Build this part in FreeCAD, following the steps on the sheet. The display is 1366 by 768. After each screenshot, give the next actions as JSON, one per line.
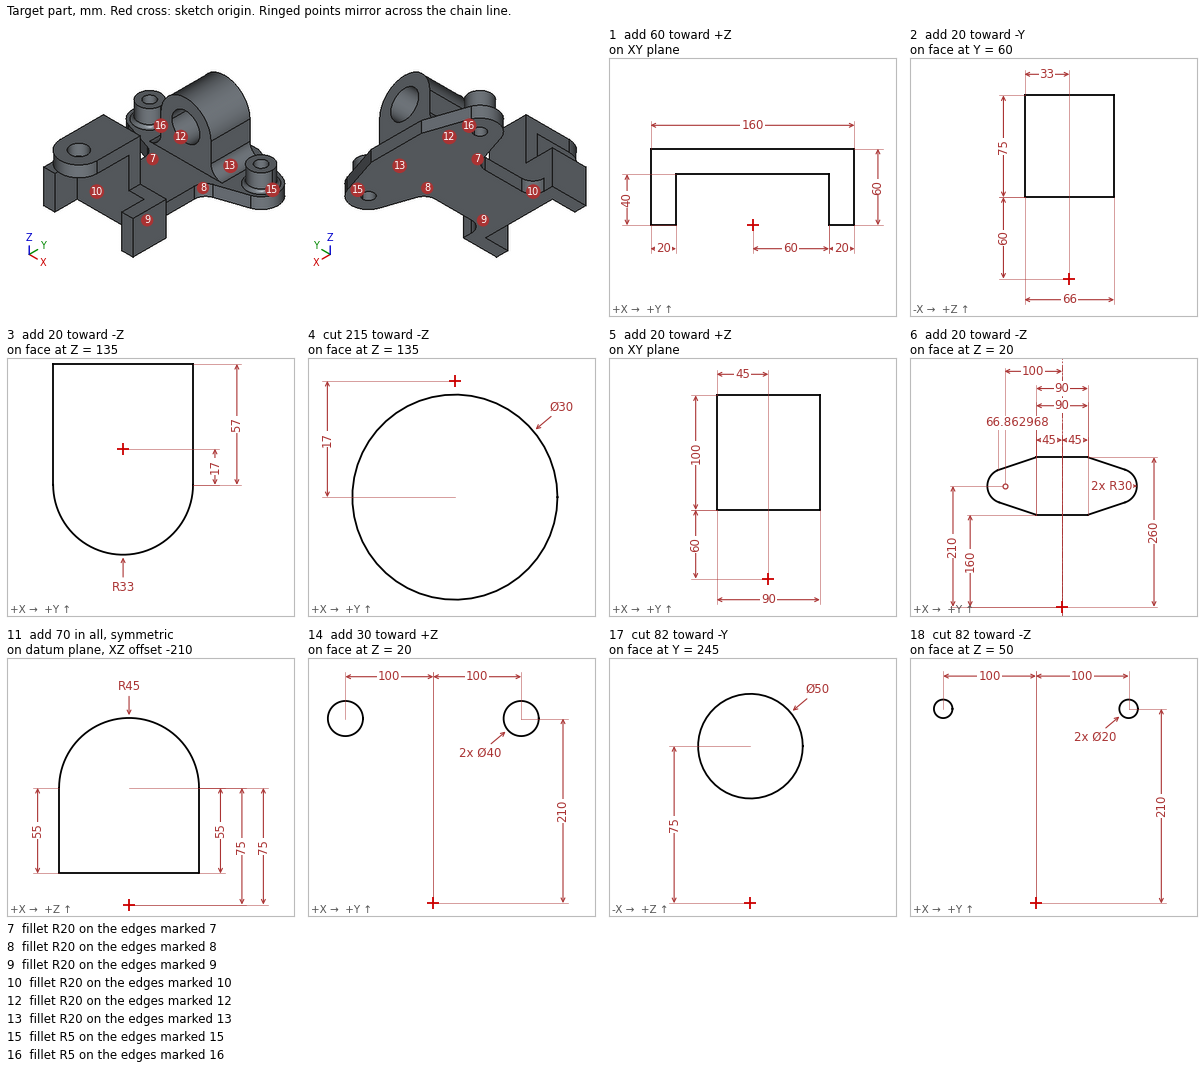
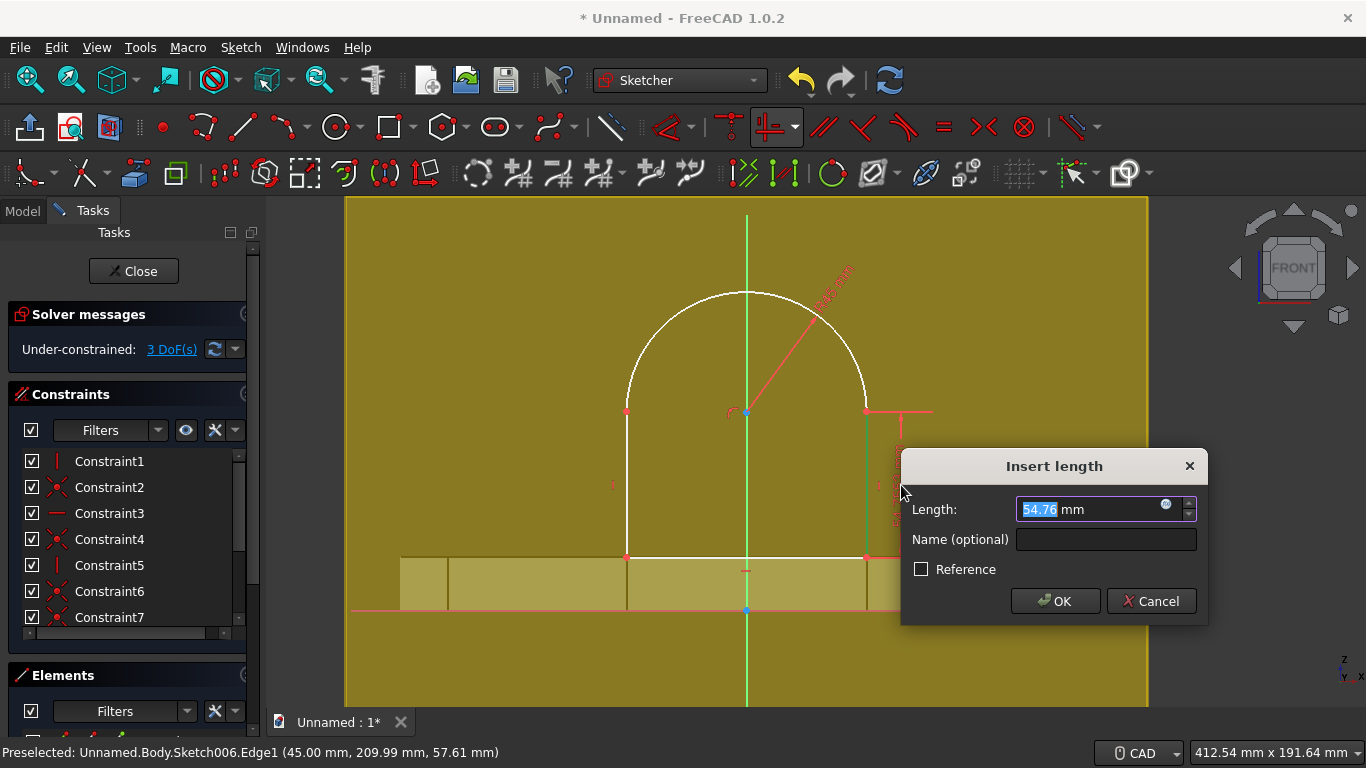
{"action": "type", "text": "55"}
{"action": "key", "text": "Return"}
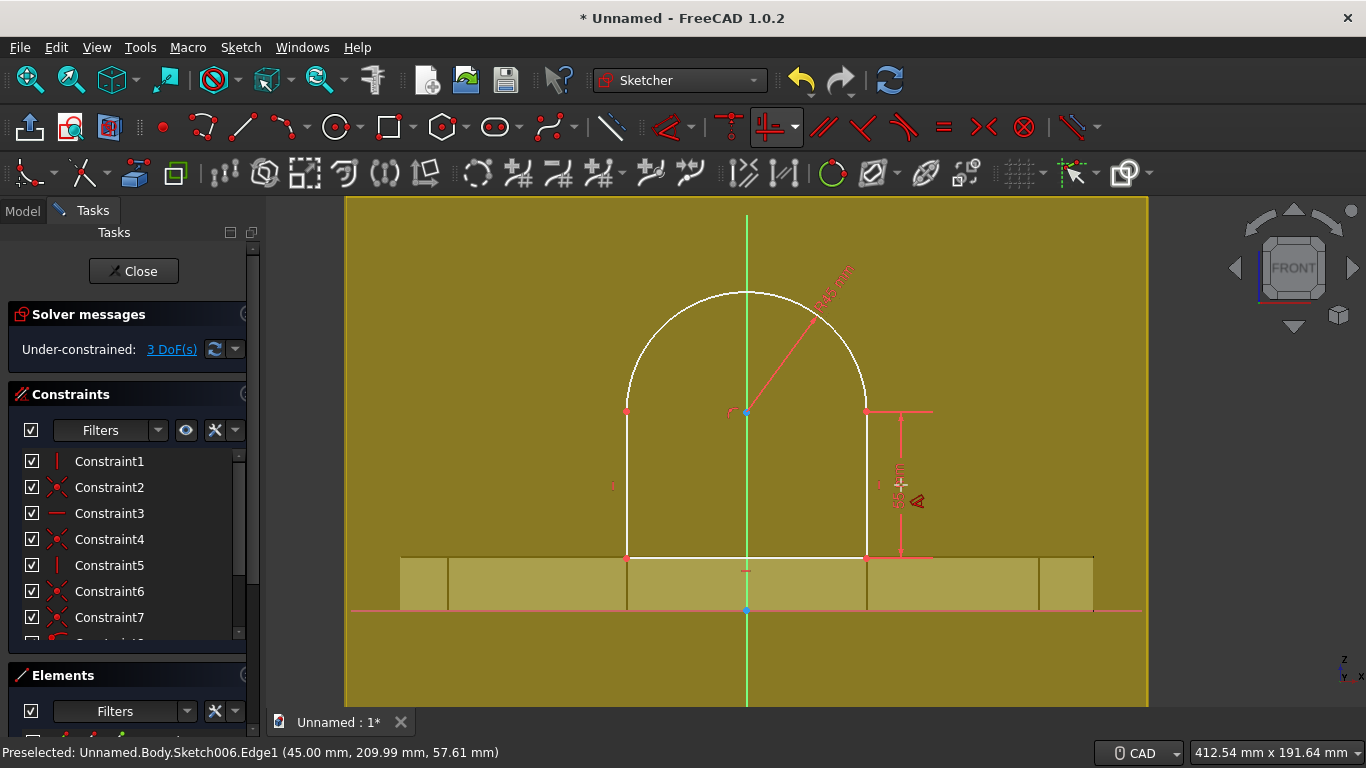
{"action": "left_click", "coordinate": [627, 514]}
{"action": "left_click", "coordinate": [593, 485]}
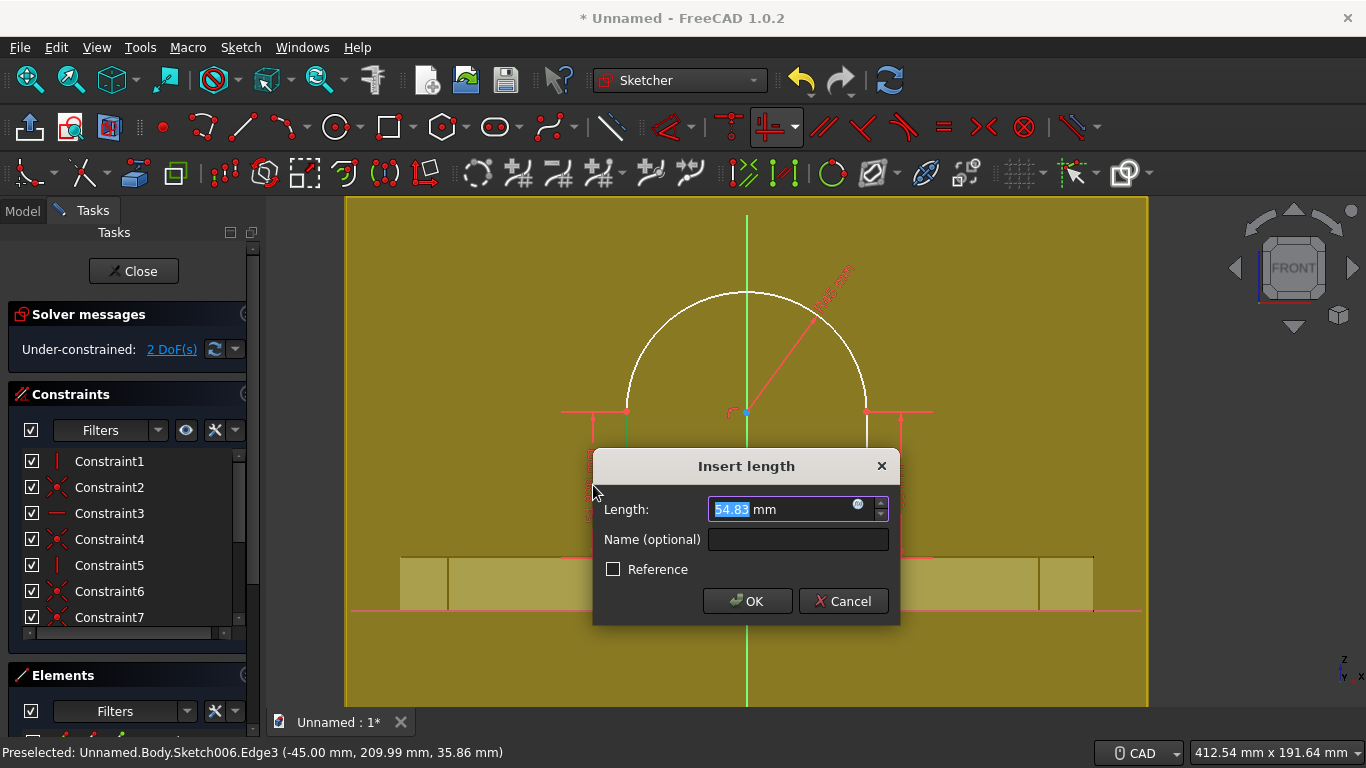
{"action": "type", "text": "55"}
{"action": "key", "text": "Return"}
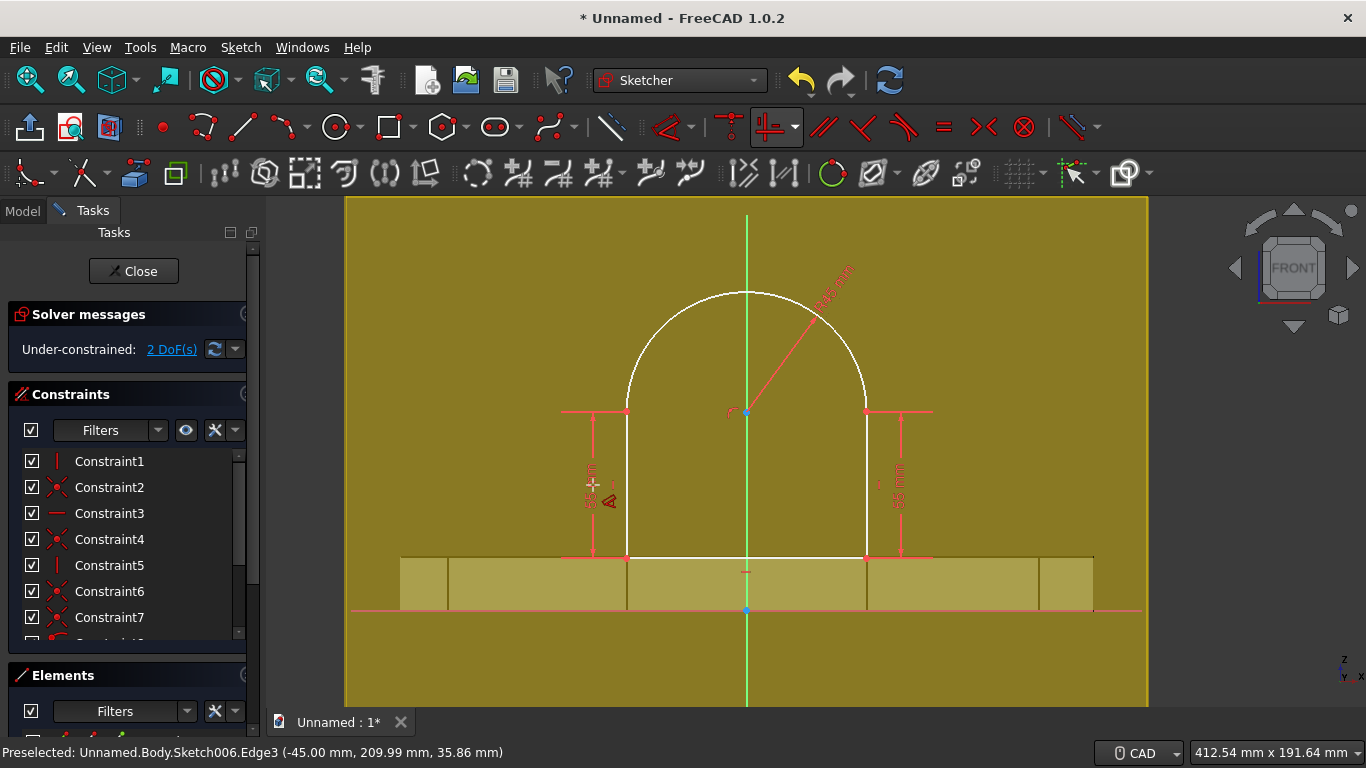
{"action": "left_click", "coordinate": [867, 412]}
{"action": "left_click", "coordinate": [901, 511]}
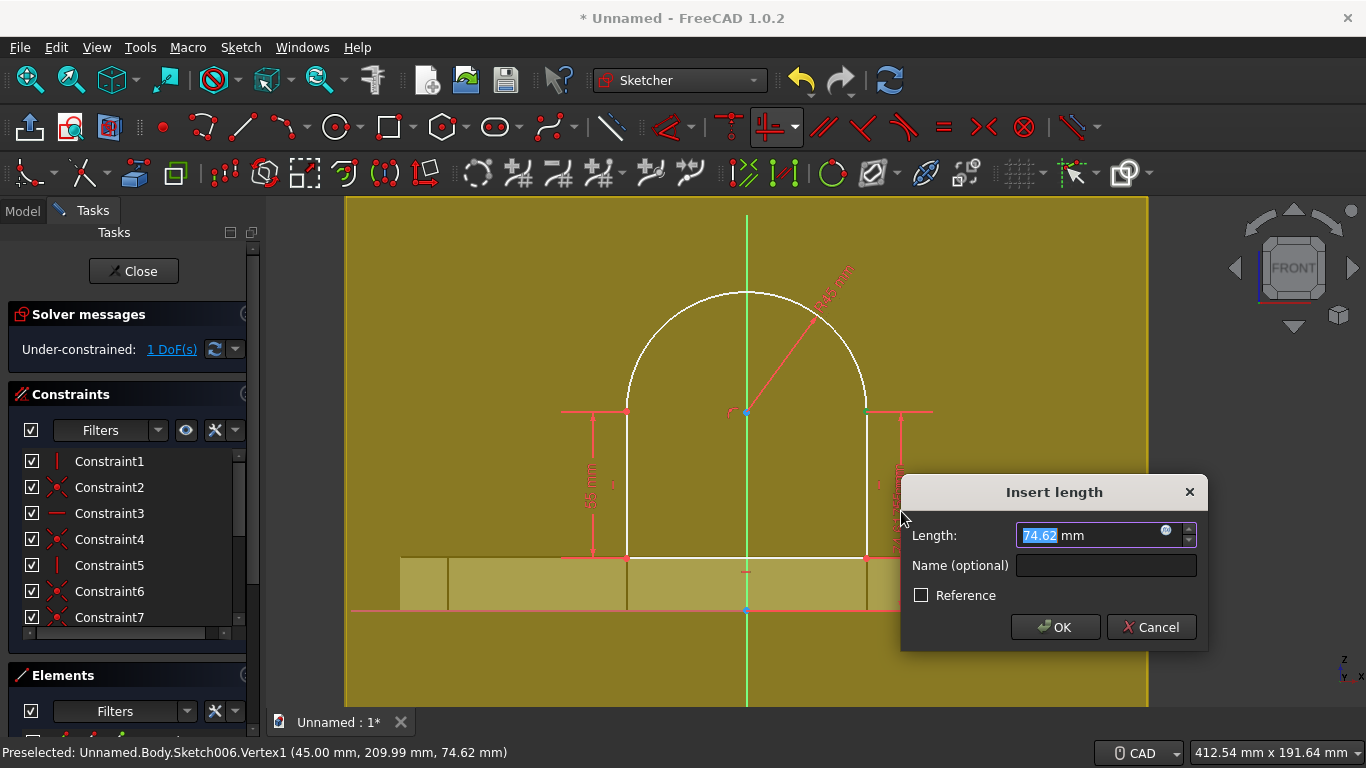
{"action": "type", "text": "75"}
{"action": "key", "text": "Return"}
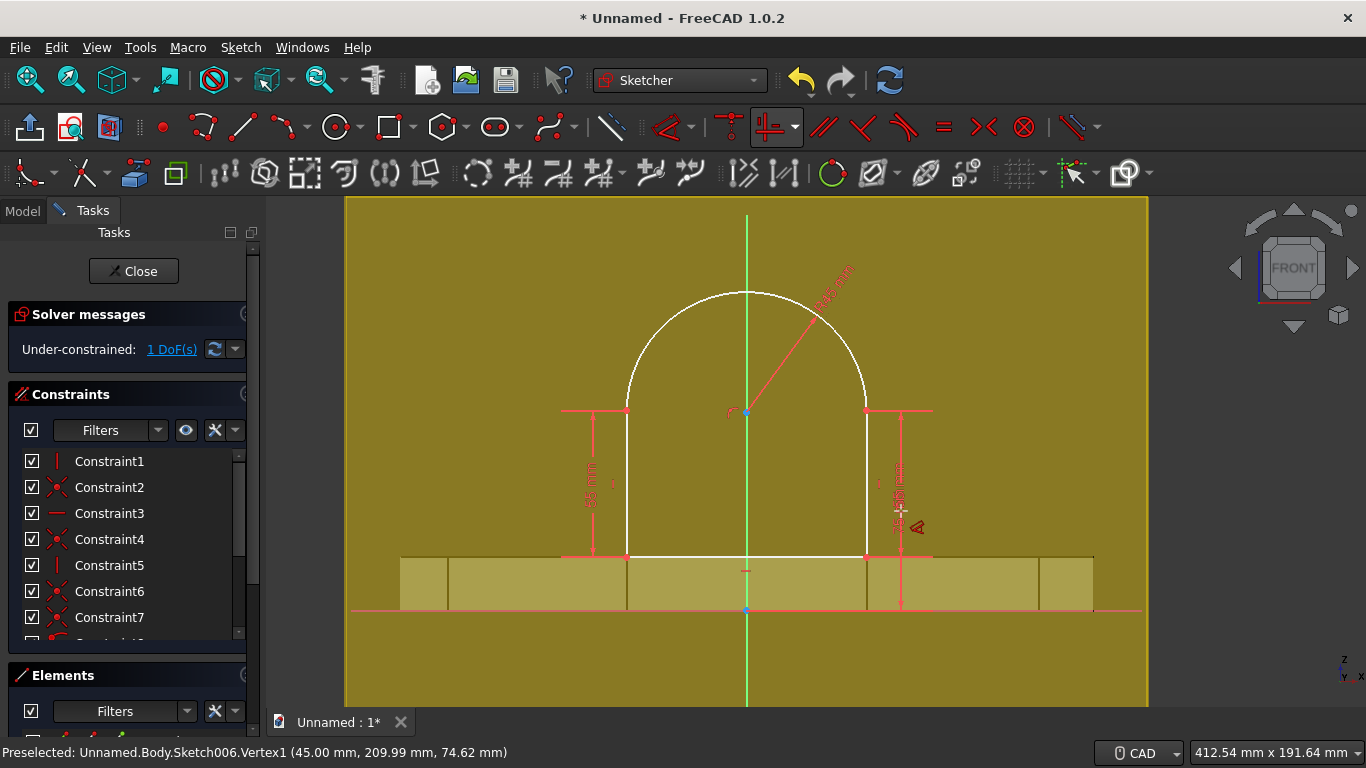
{"action": "left_click", "coordinate": [747, 412]}
{"action": "left_click", "coordinate": [781, 511]}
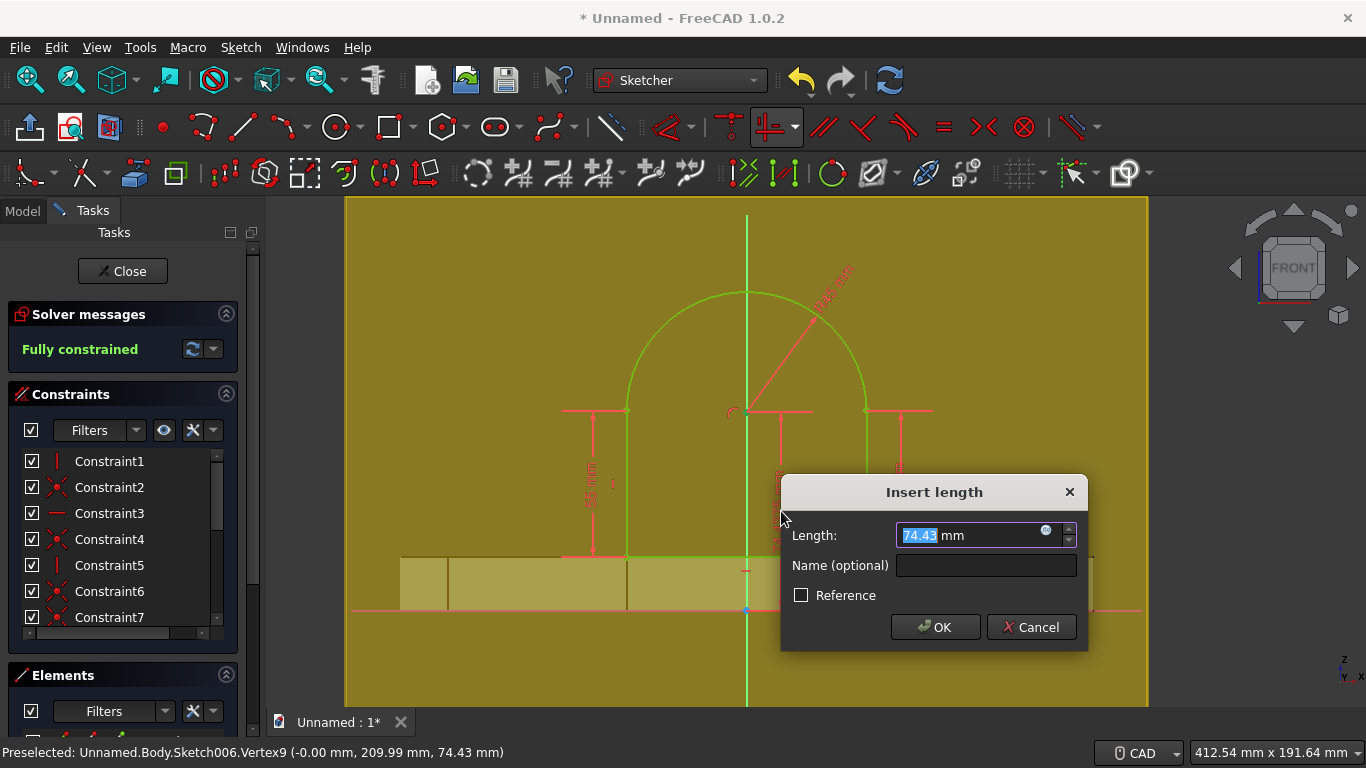
{"action": "type", "text": "75"}
{"action": "key", "text": "Return"}
{"action": "key", "text": "Escape"}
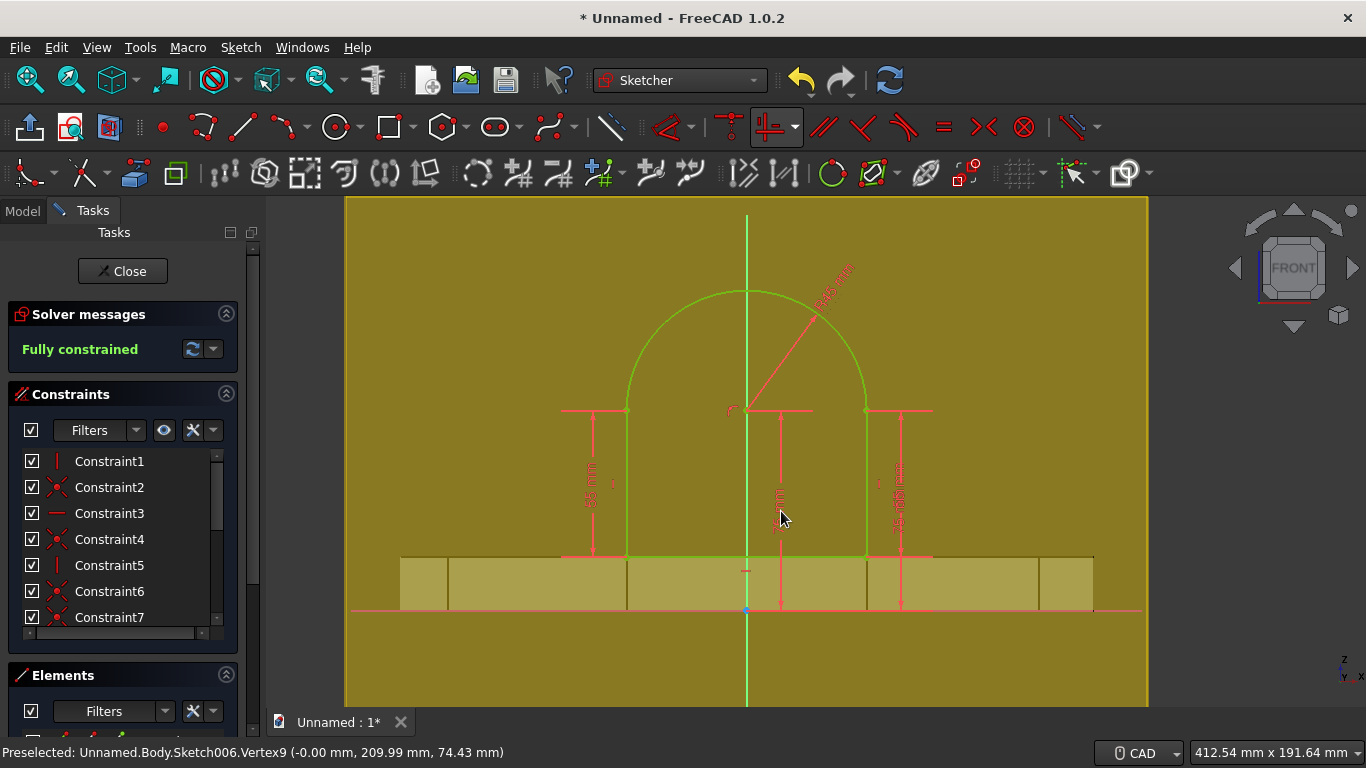
{"action": "left_click", "coordinate": [123, 271]}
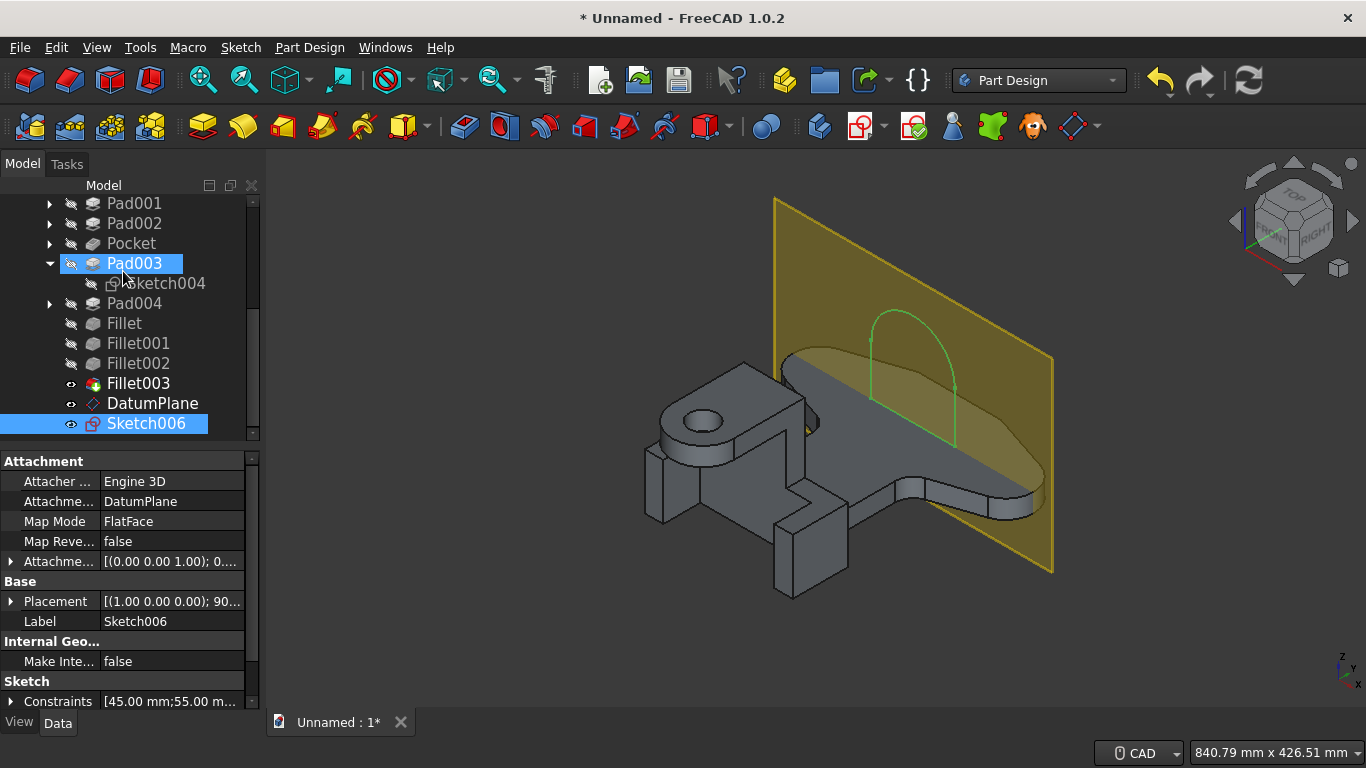
{"action": "left_click", "coordinate": [204, 126]}